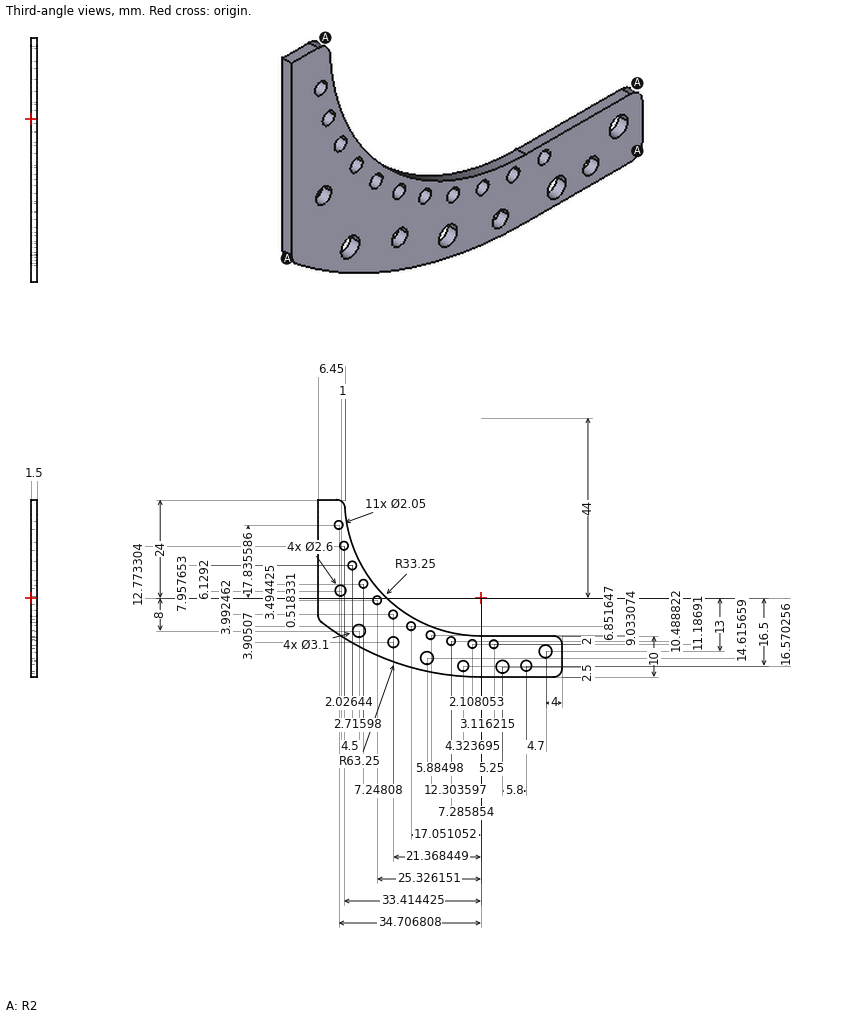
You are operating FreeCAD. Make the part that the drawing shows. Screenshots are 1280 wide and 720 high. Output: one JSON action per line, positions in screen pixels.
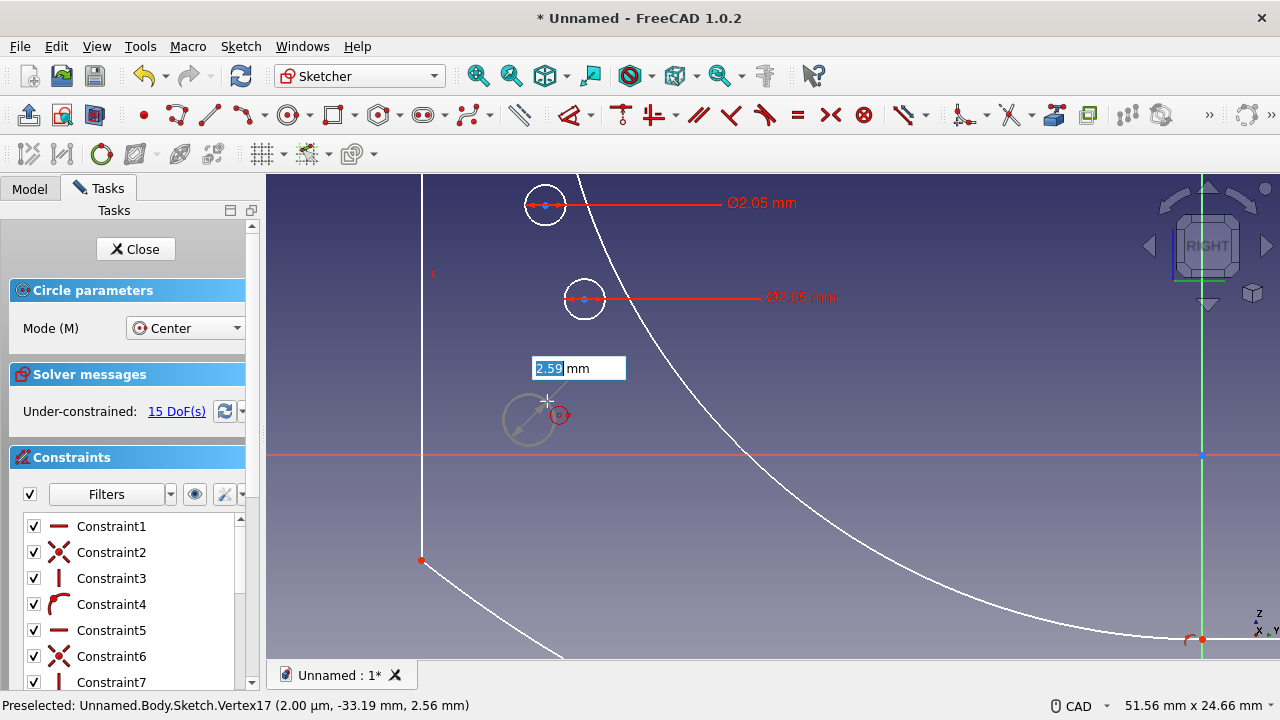
{"action": "type", "text": "2.6"}
{"action": "key", "text": "Return"}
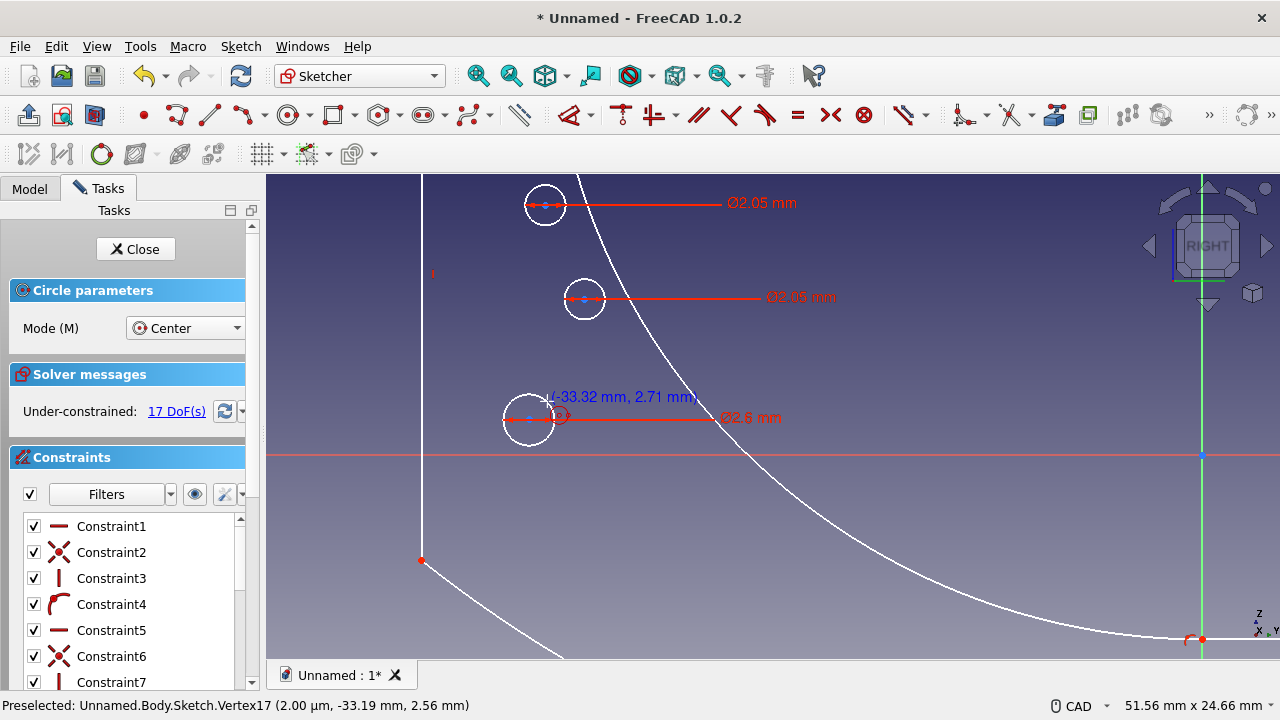
{"action": "left_click", "coordinate": [639, 387]}
{"action": "mouse_move", "coordinate": [653, 372]}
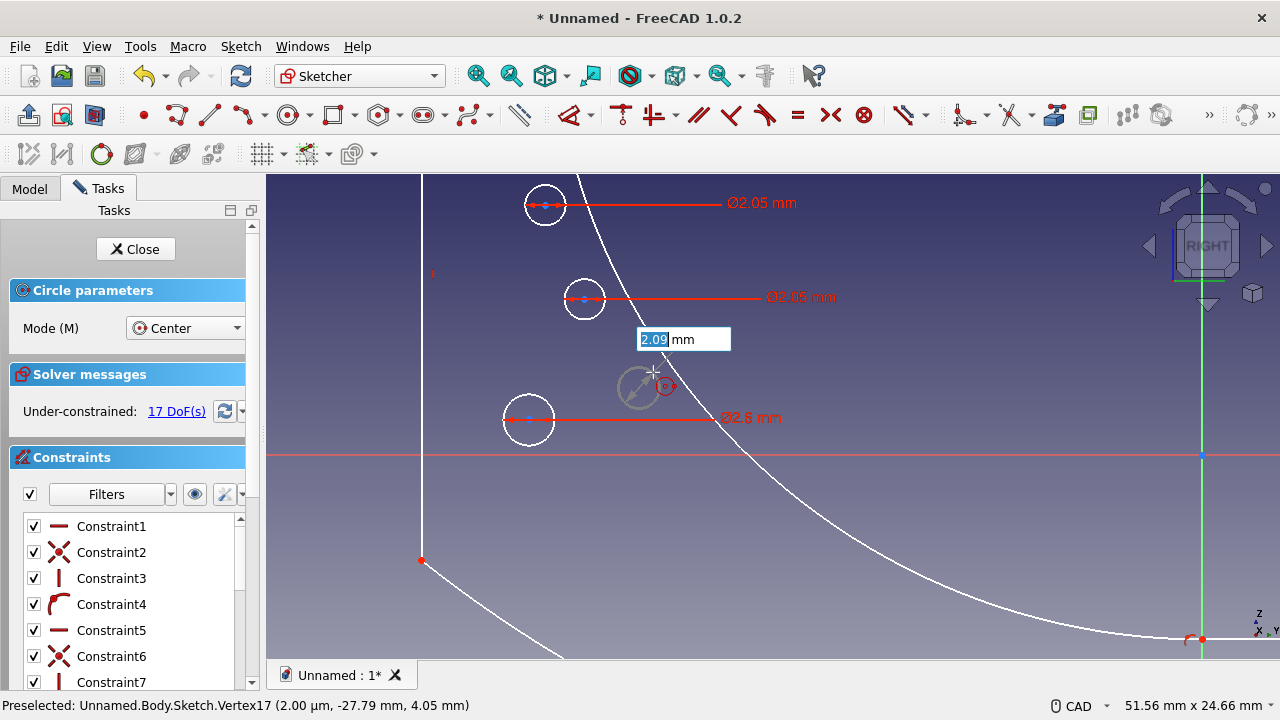
{"action": "type", "text": "2.05"}
{"action": "key", "text": "Return"}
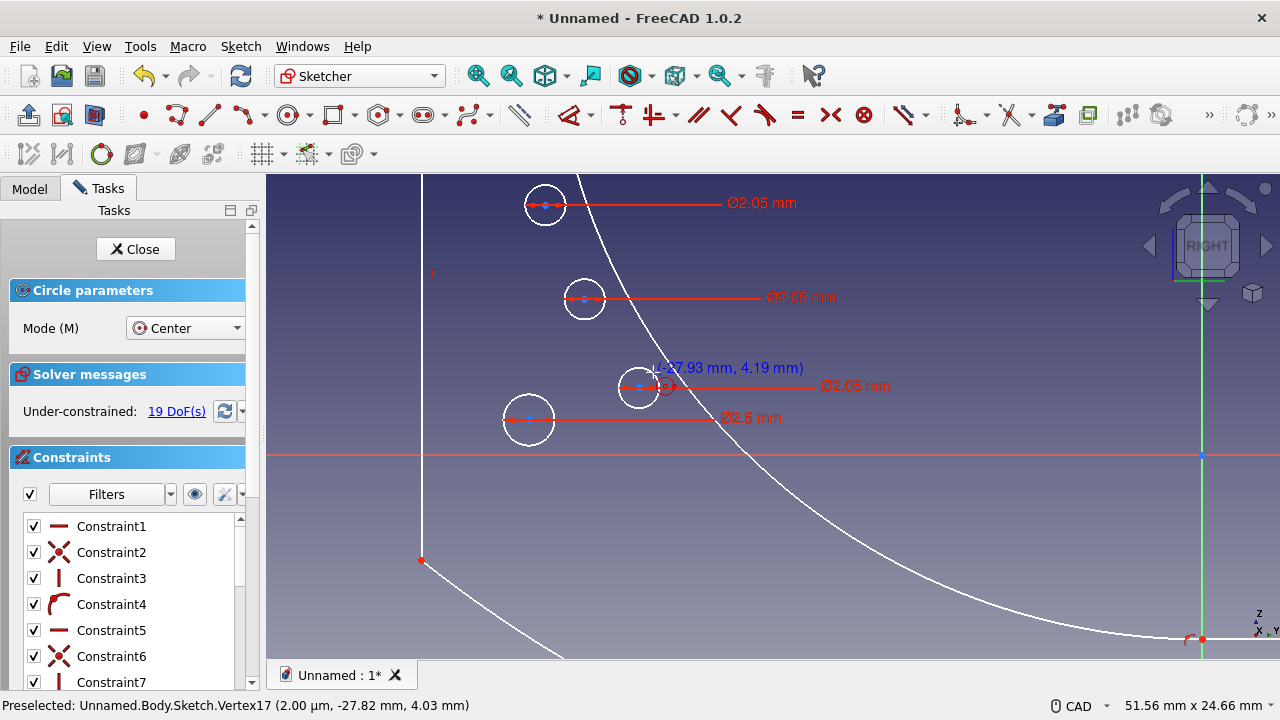
{"action": "left_click", "coordinate": [617, 613]}
{"action": "mouse_move", "coordinate": [639, 591]}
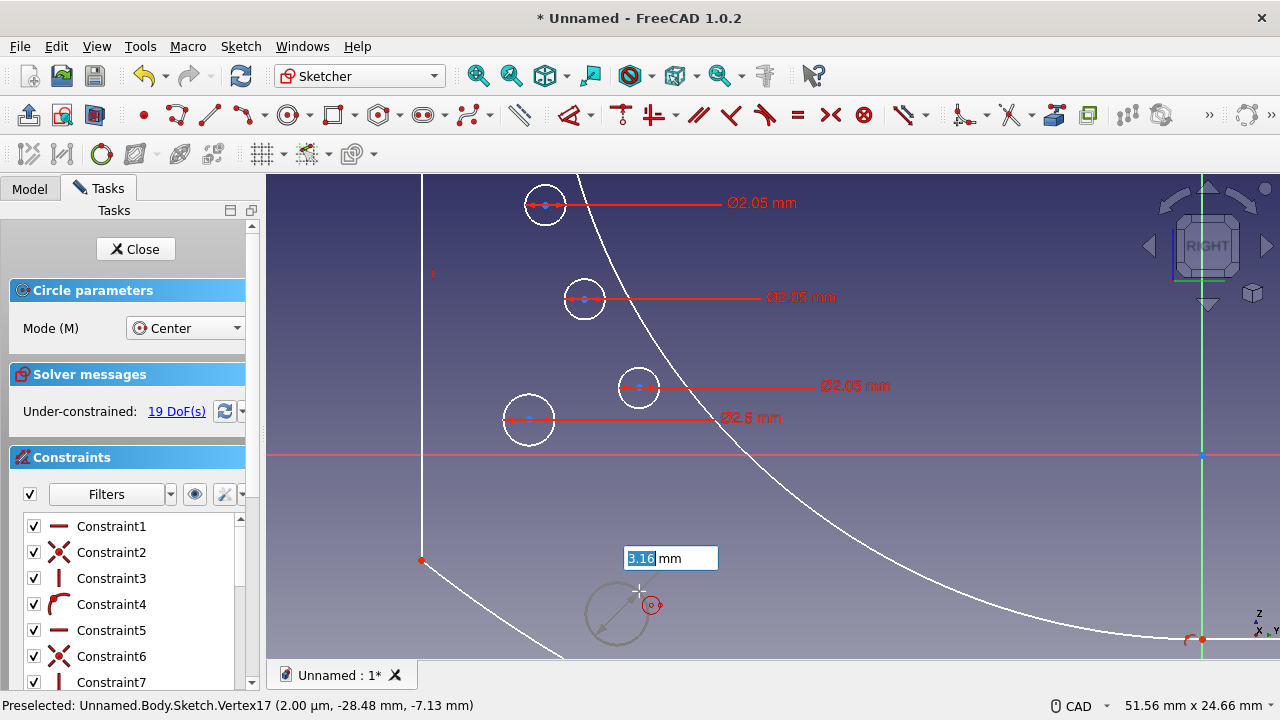
{"action": "type", "text": "3.1"}
{"action": "key", "text": "Return"}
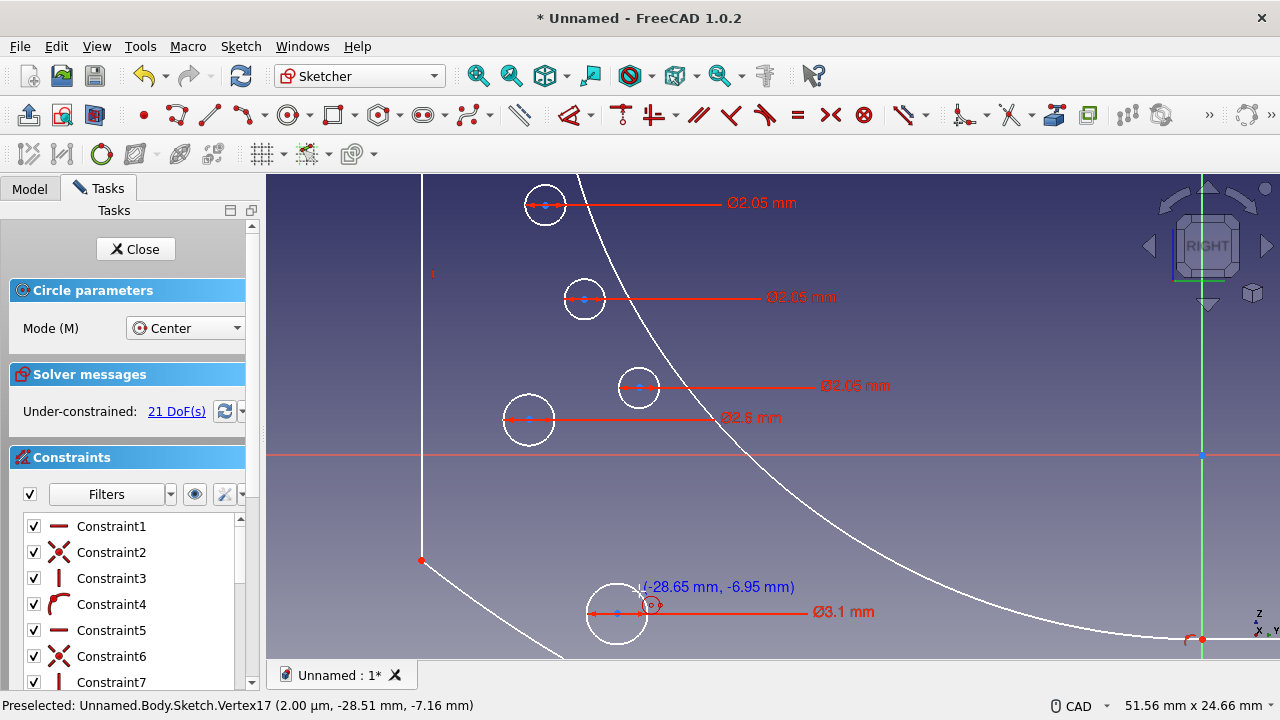
{"action": "scroll", "coordinate": [704, 466], "scroll_direction": "up", "scroll_amount": 3}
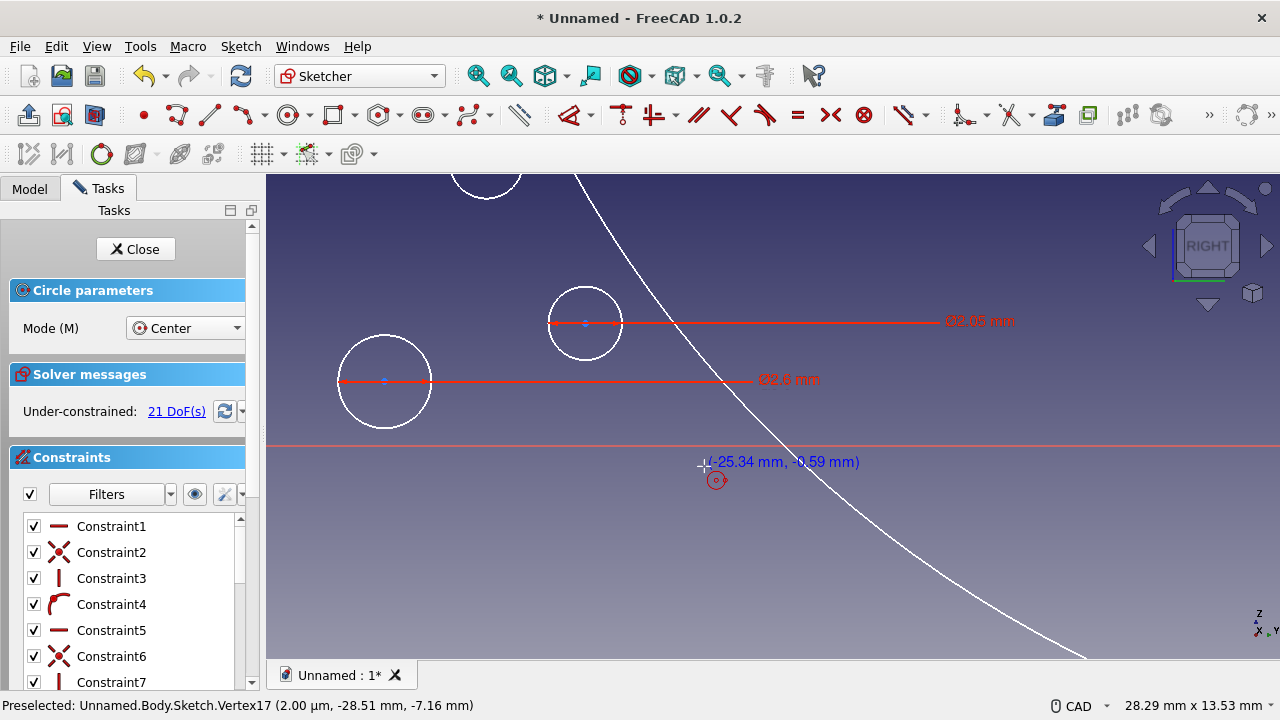
{"action": "left_click", "coordinate": [704, 465]}
{"action": "mouse_move", "coordinate": [730, 491]}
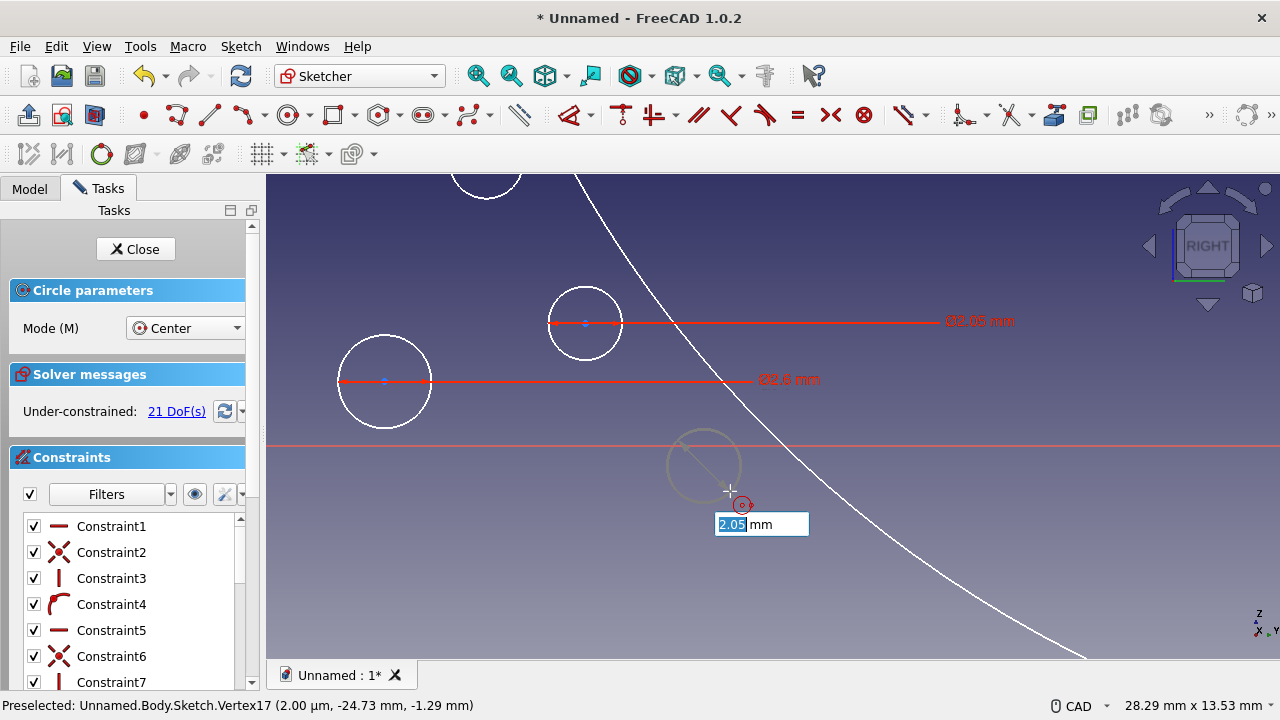
{"action": "type", "text": "2.05"}
{"action": "key", "text": "Return"}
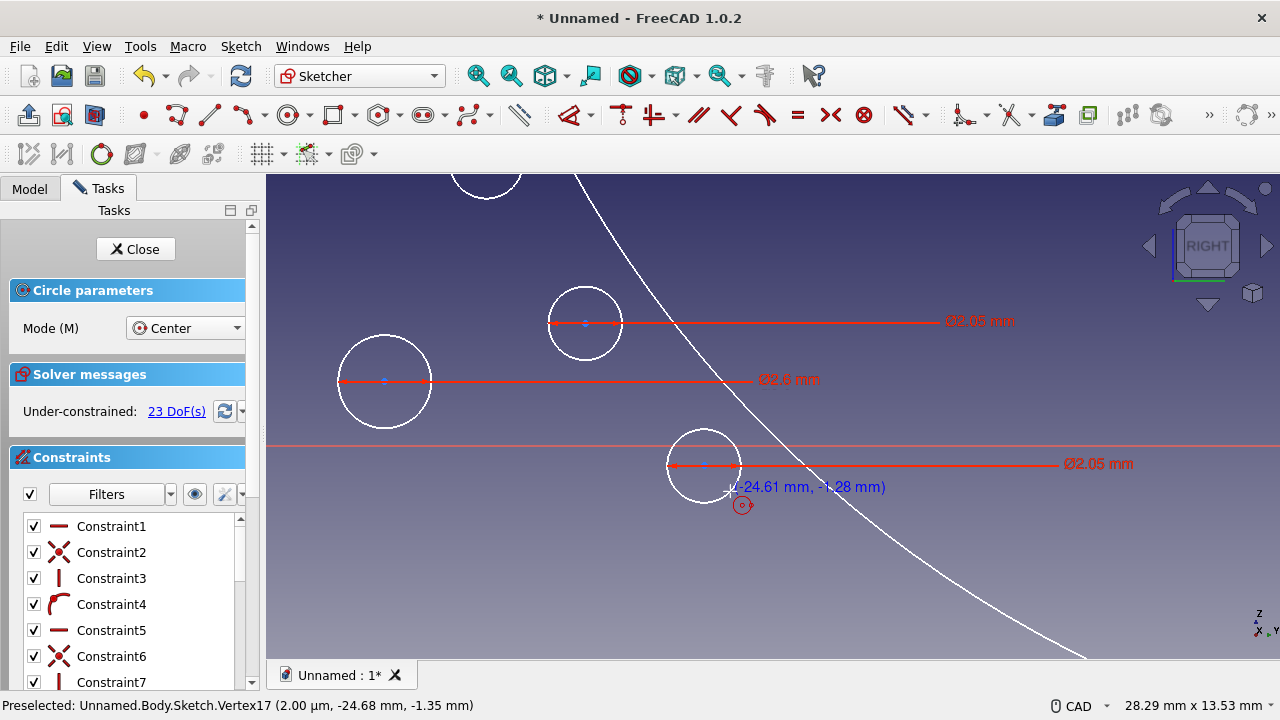
{"action": "scroll", "coordinate": [565, 431], "scroll_direction": "down", "scroll_amount": 8}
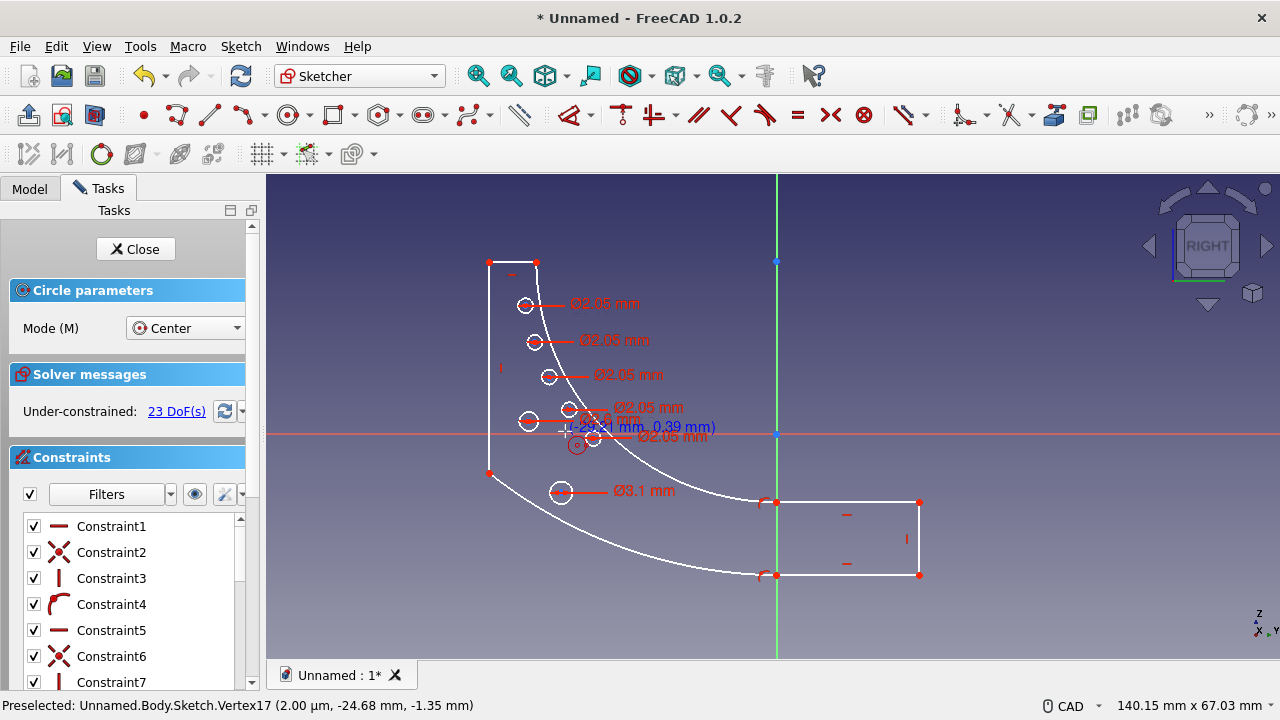
{"action": "left_click", "coordinate": [622, 463]}
{"action": "mouse_move", "coordinate": [627, 469]}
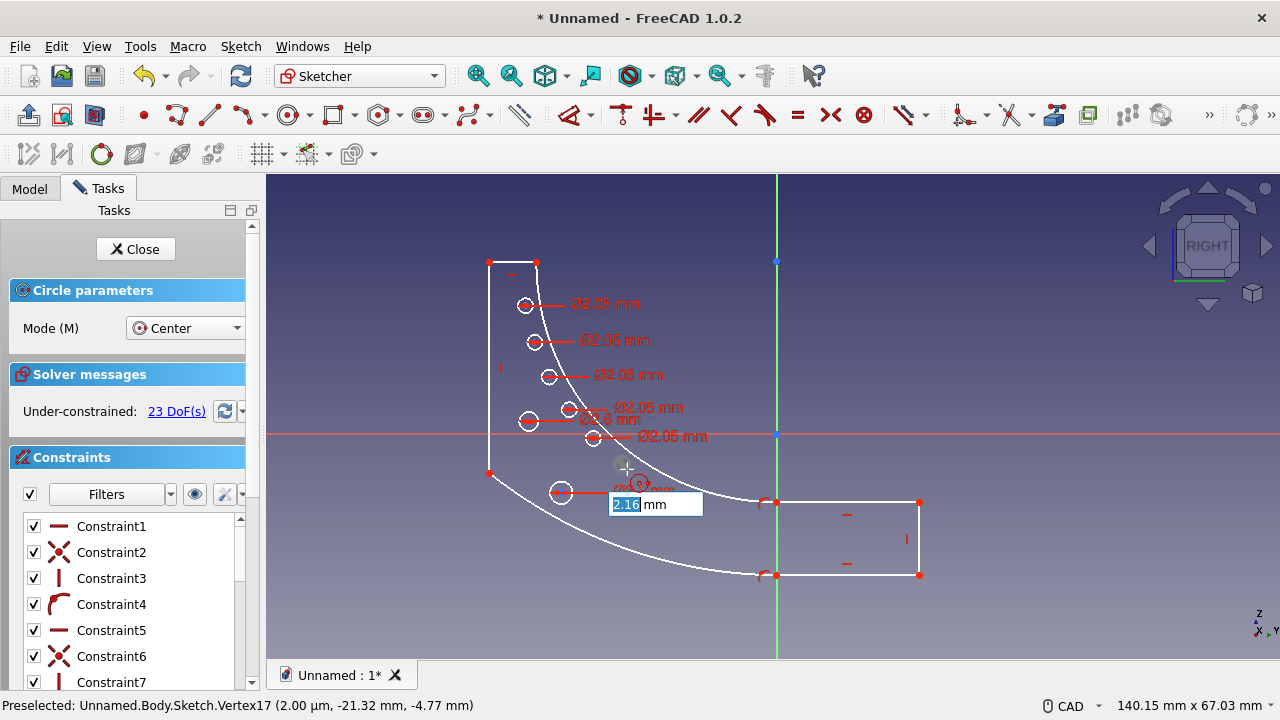
{"action": "type", "text": "2.05"}
{"action": "key", "text": "Return"}